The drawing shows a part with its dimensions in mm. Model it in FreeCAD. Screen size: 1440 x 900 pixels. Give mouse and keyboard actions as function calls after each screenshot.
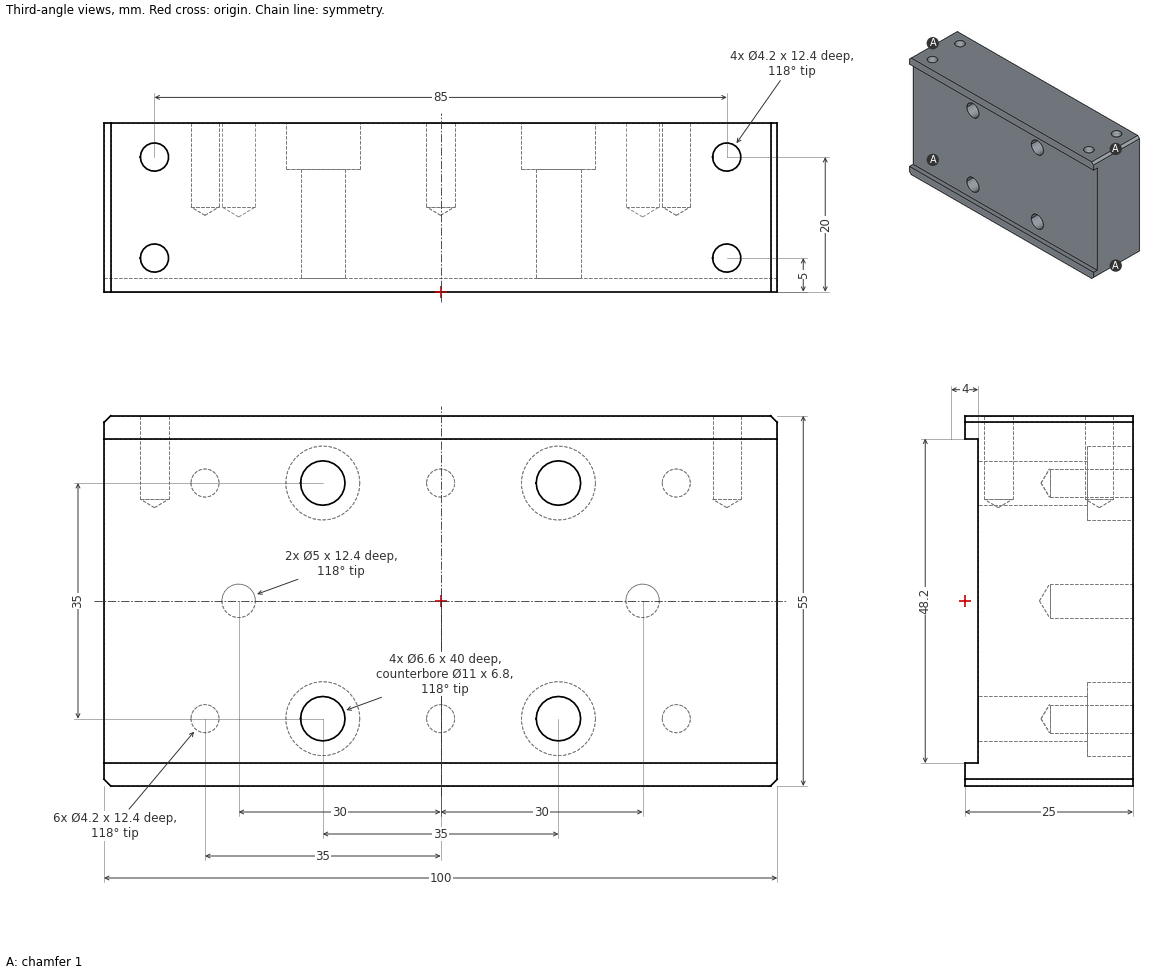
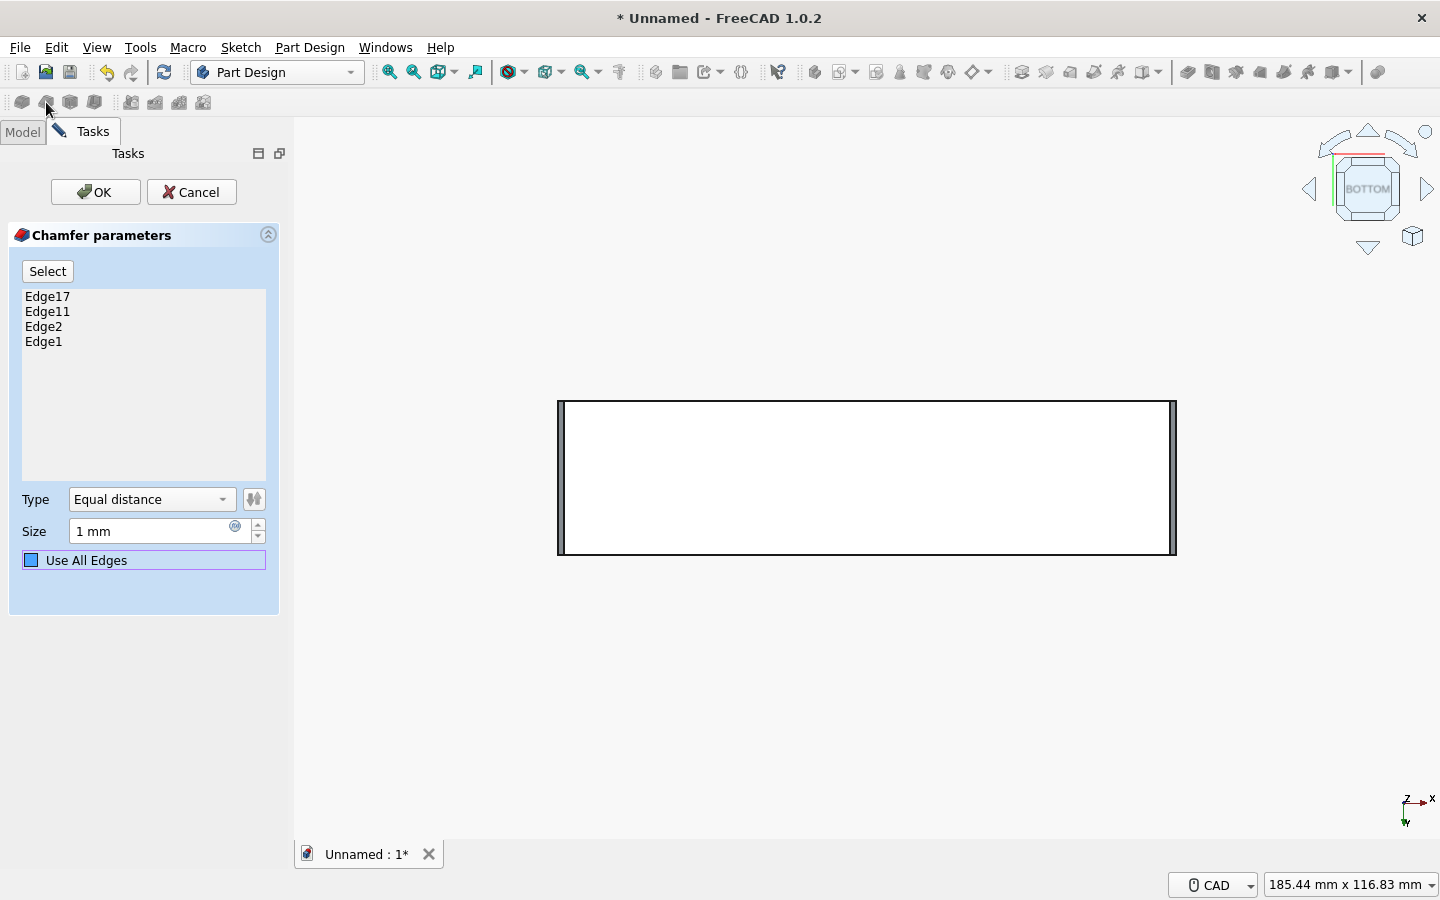
click(96, 192)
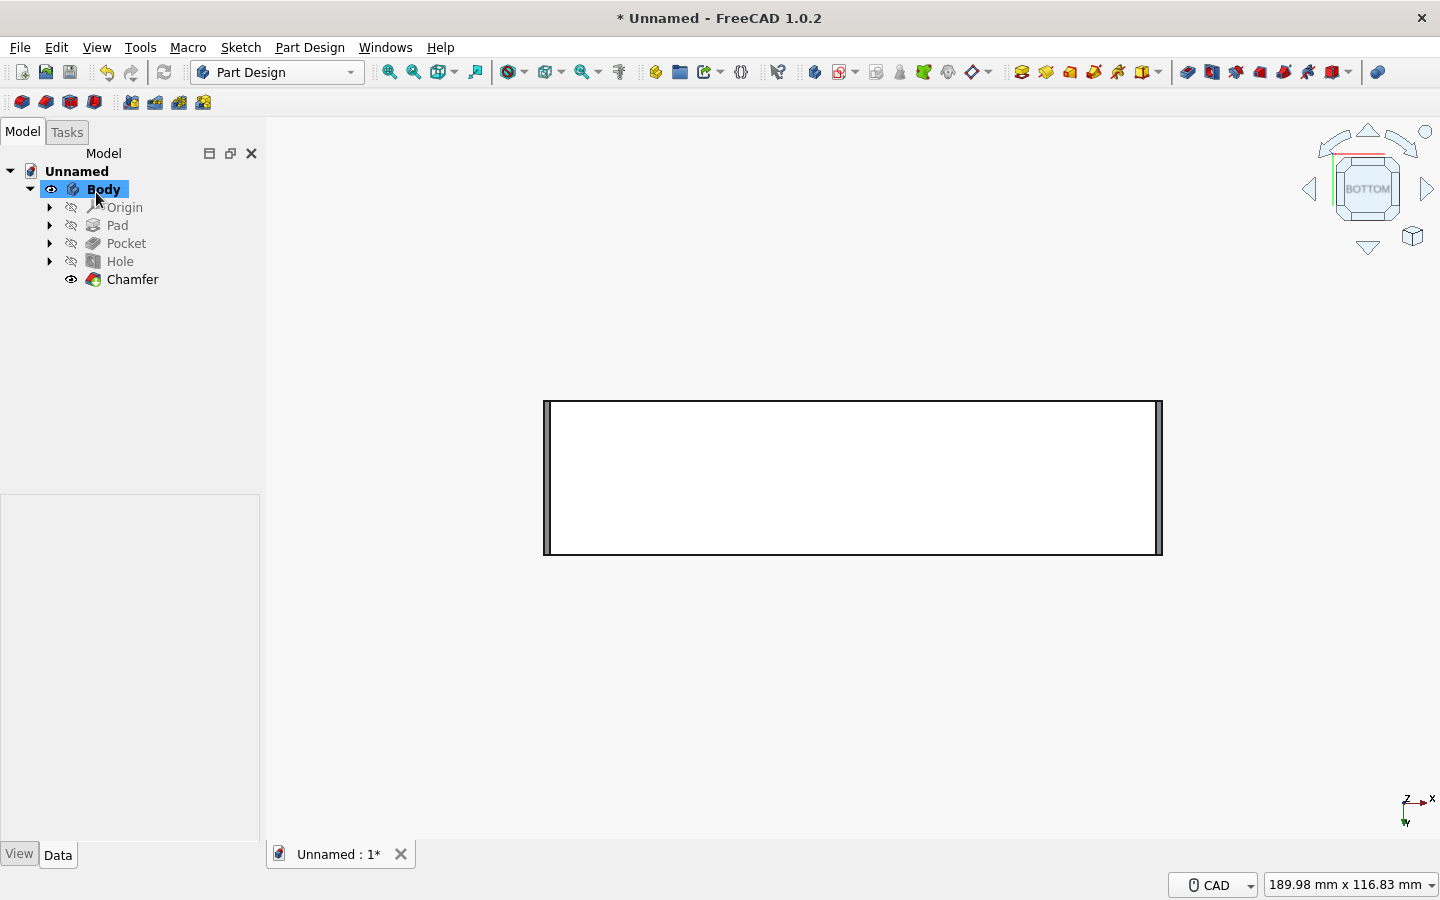
key(4)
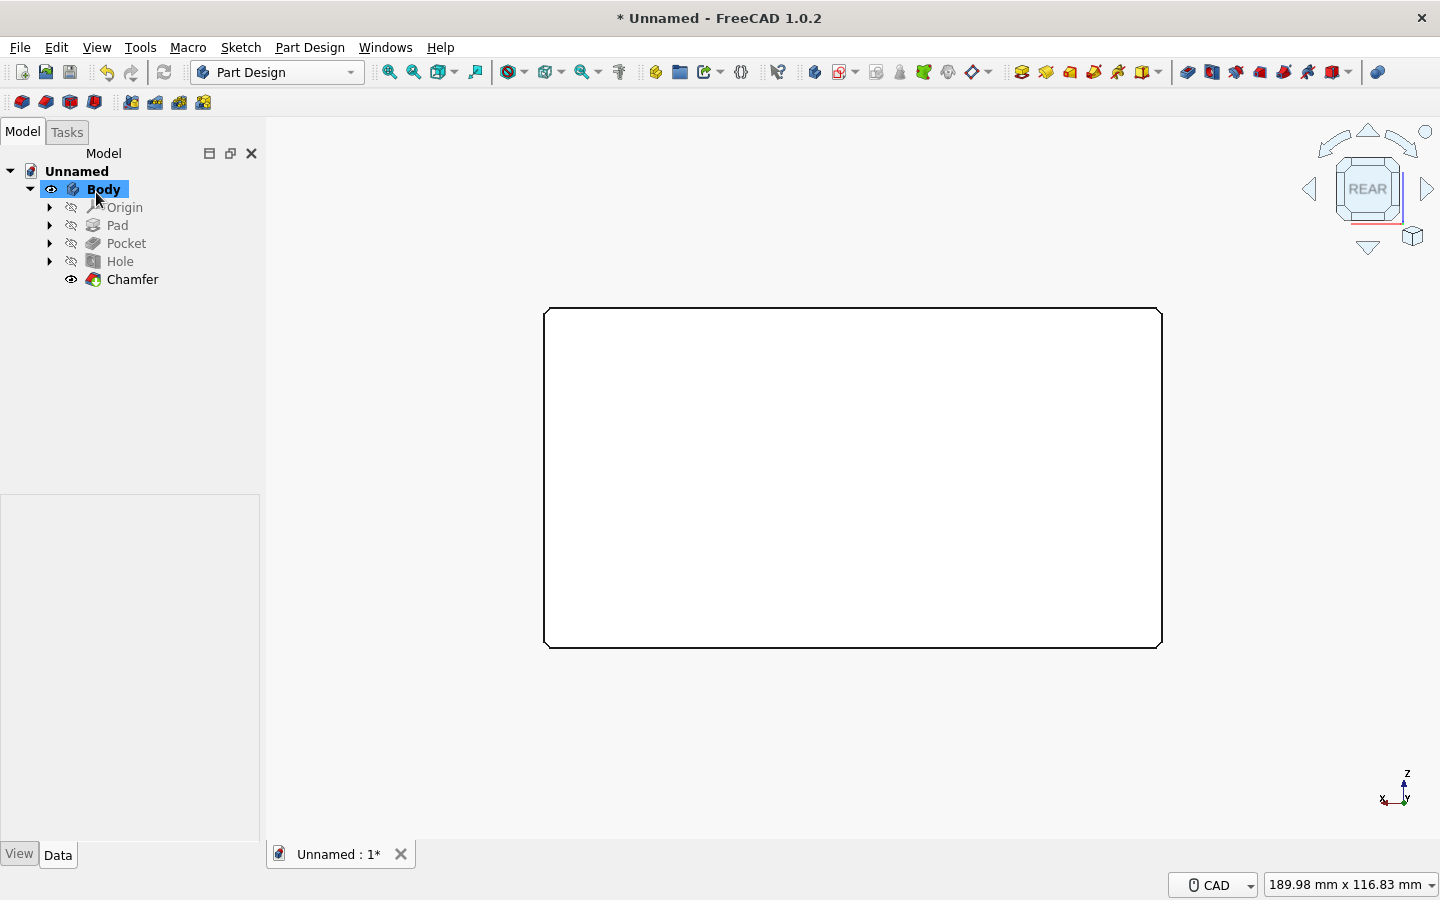
click(765, 477)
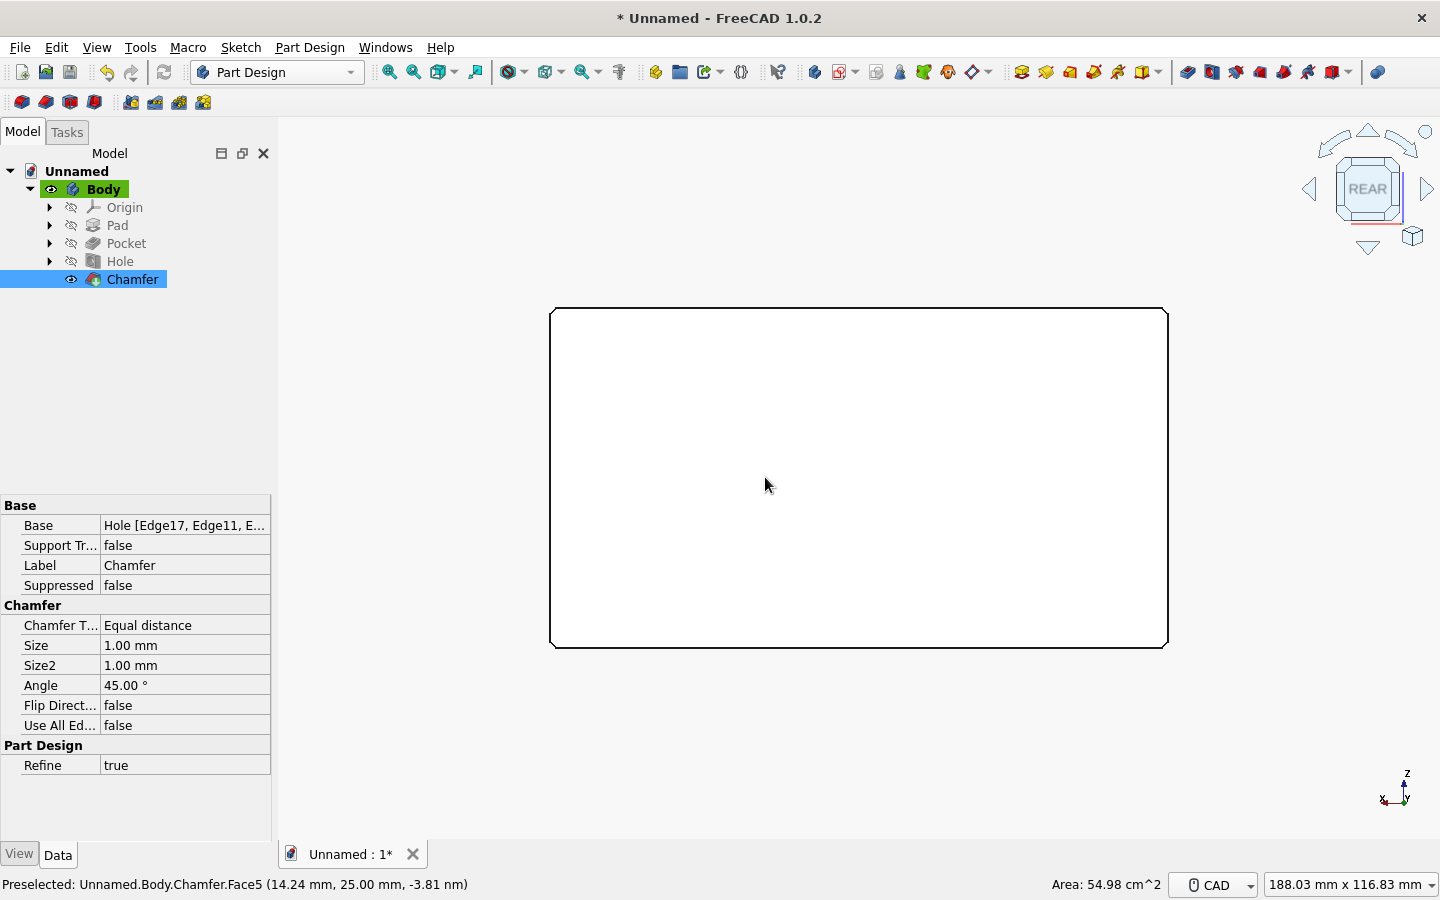
click(840, 72)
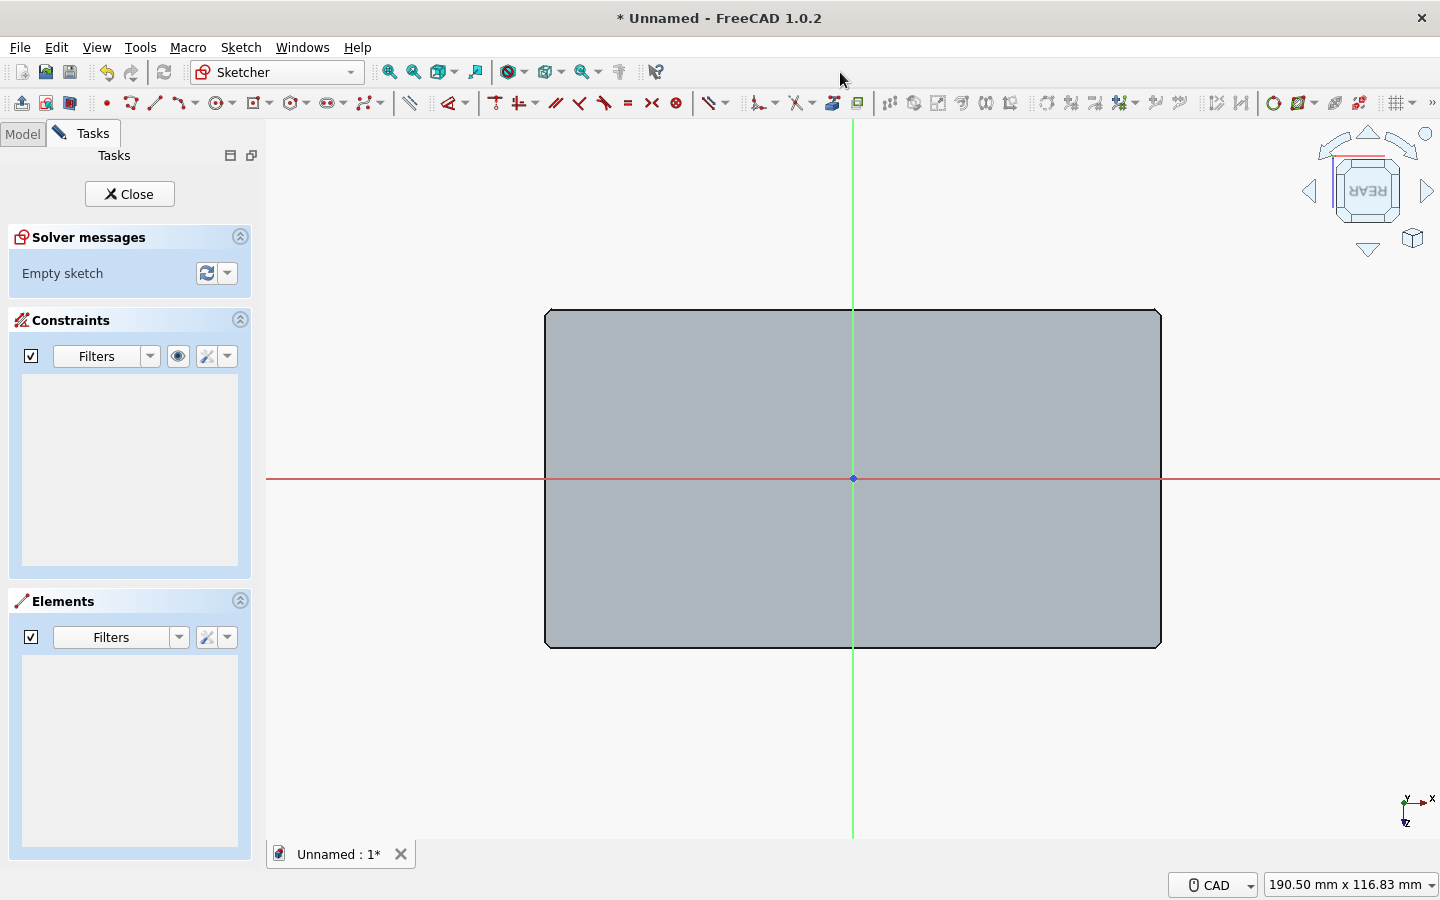
scroll(936, 479, up, 3)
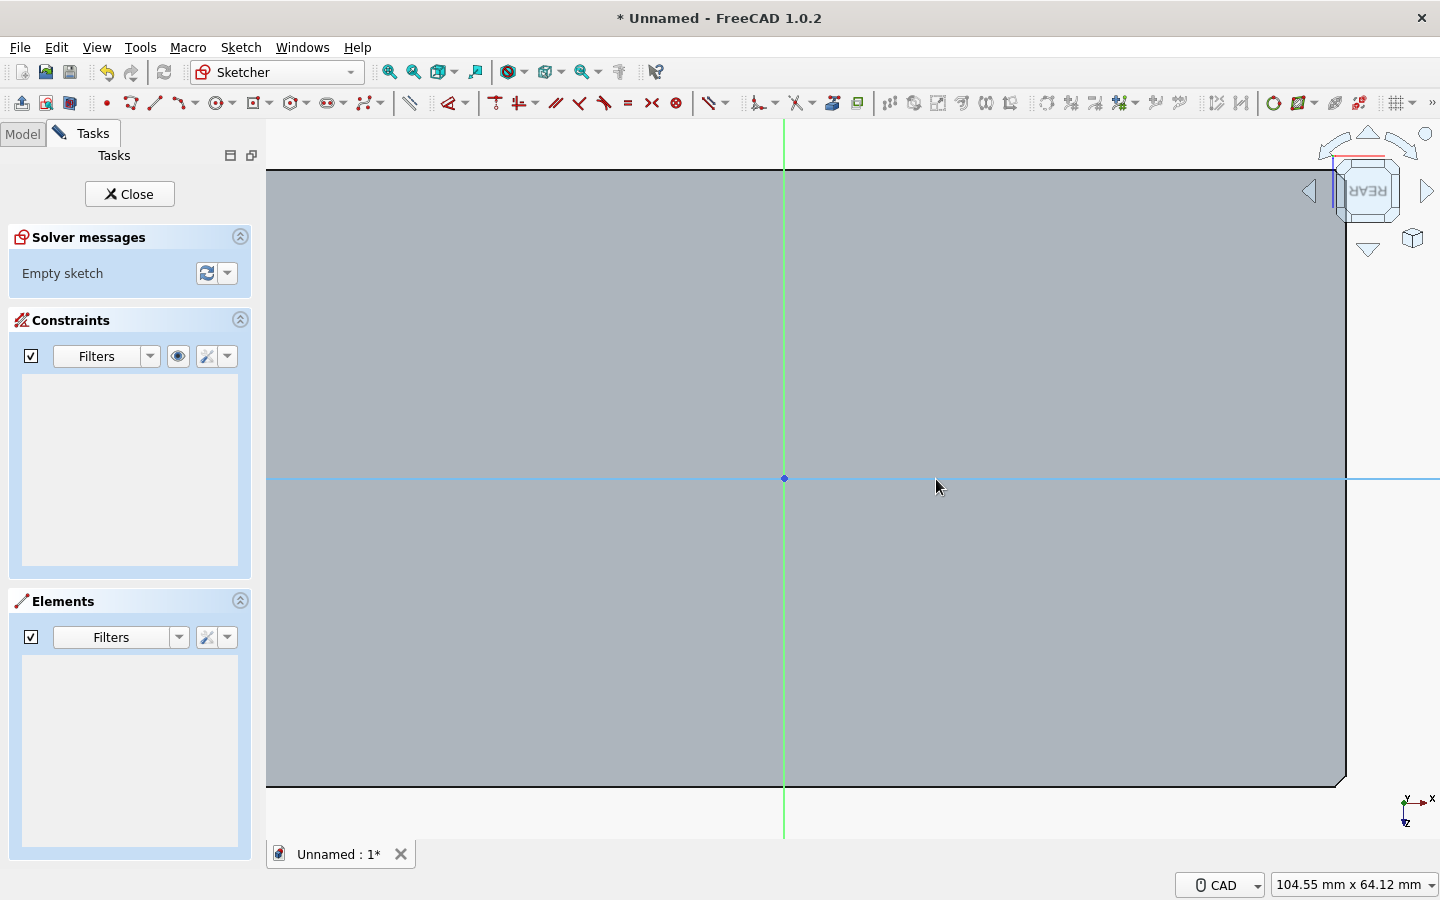
click(216, 104)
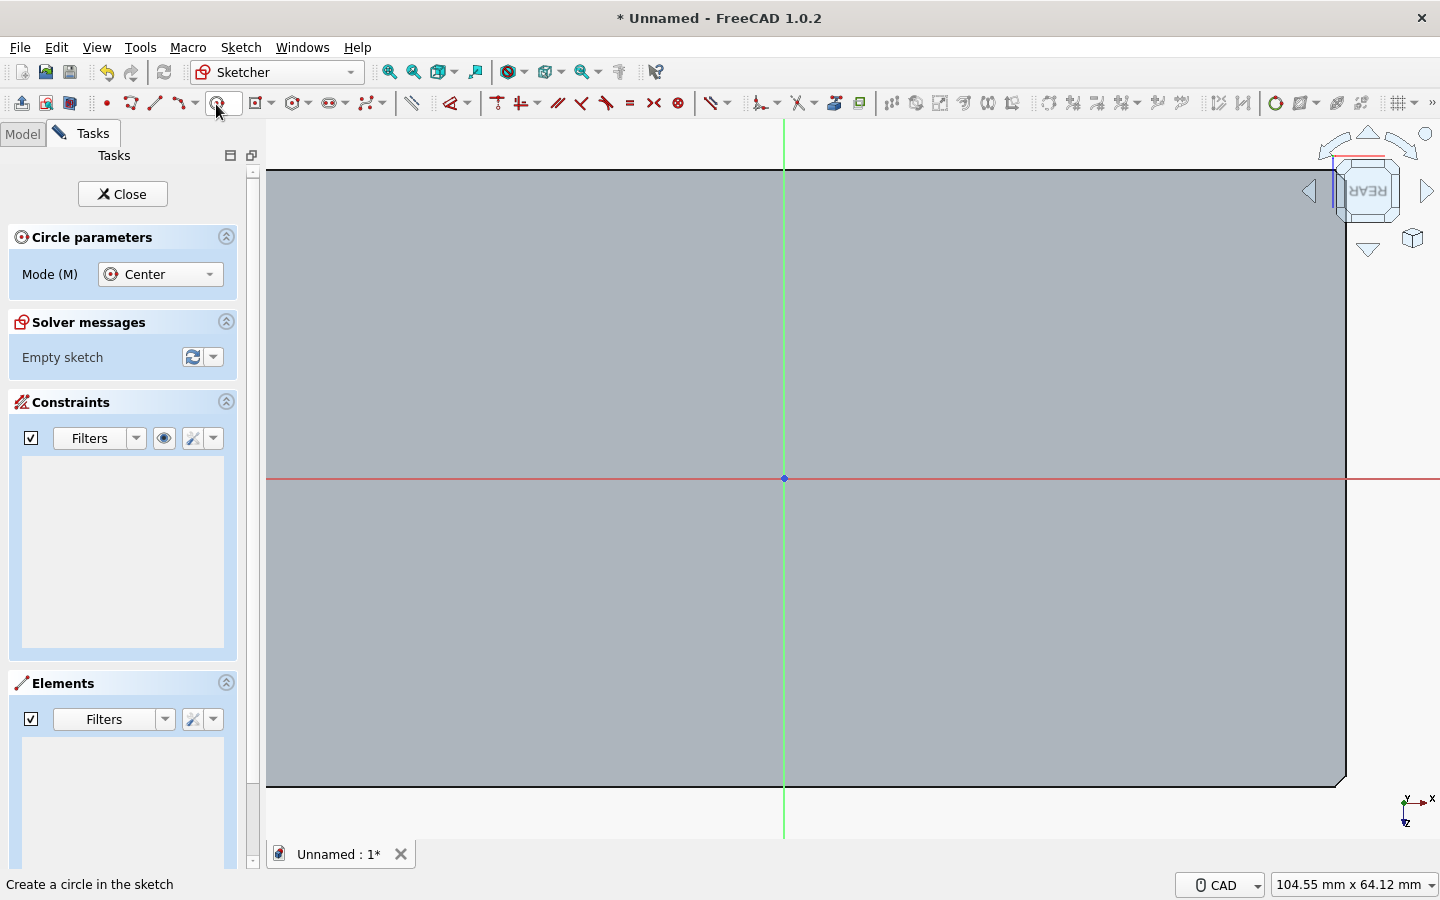
click(588, 282)
move(614, 256)